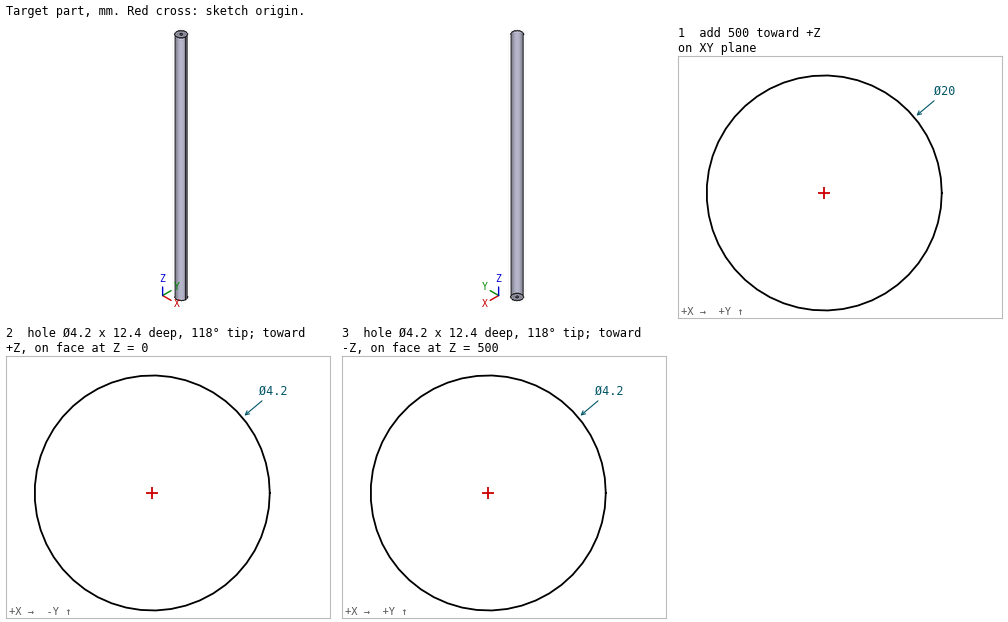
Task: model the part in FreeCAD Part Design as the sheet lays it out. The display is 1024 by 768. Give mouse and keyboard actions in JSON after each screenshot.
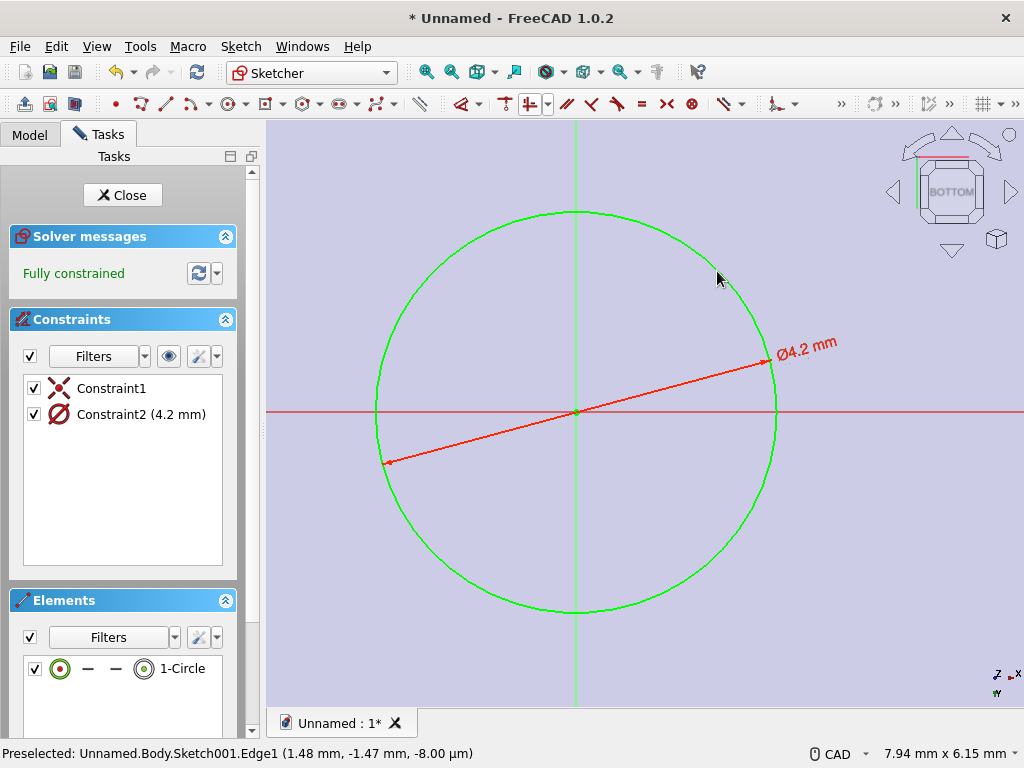
{"action": "left_click", "coordinate": [123, 195]}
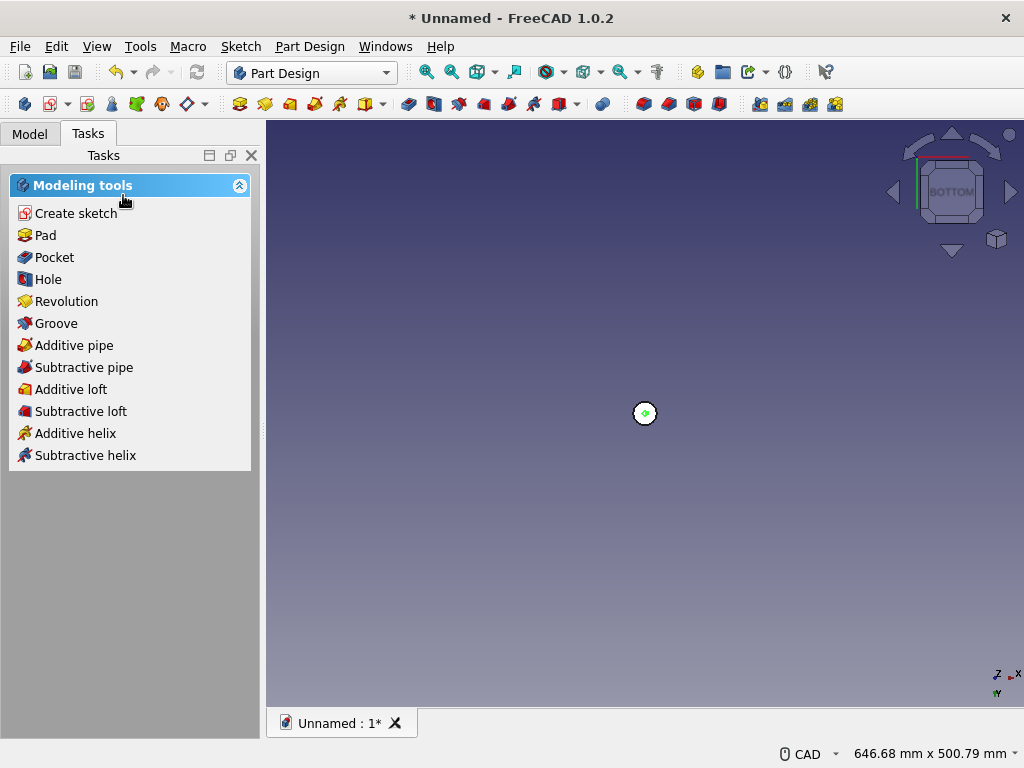
{"action": "left_click", "coordinate": [434, 104]}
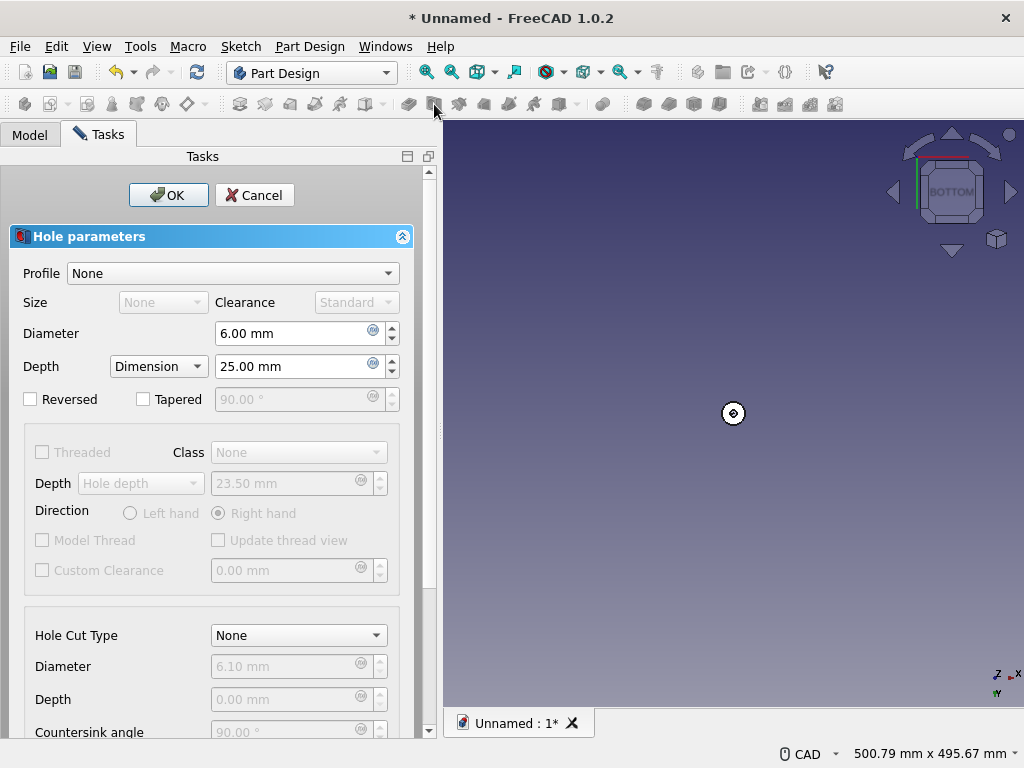
{"action": "triple_click", "coordinate": [300, 334]}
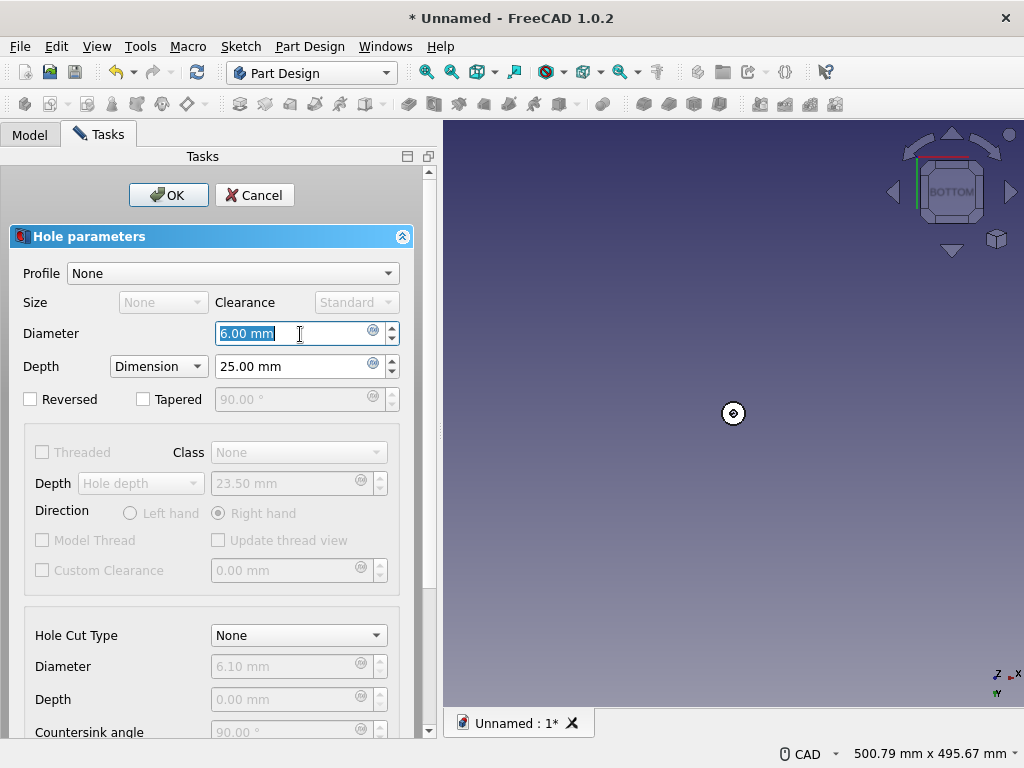
{"action": "type", "text": "4.2"}
{"action": "key", "text": "Tab"}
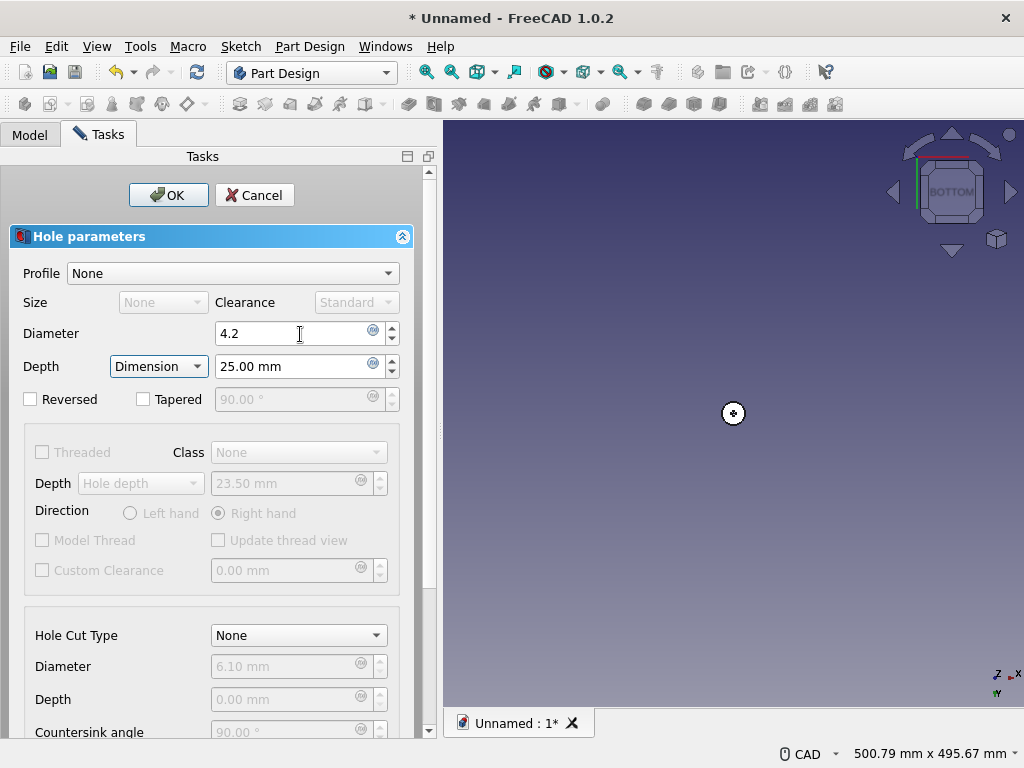
{"action": "triple_click", "coordinate": [300, 366]}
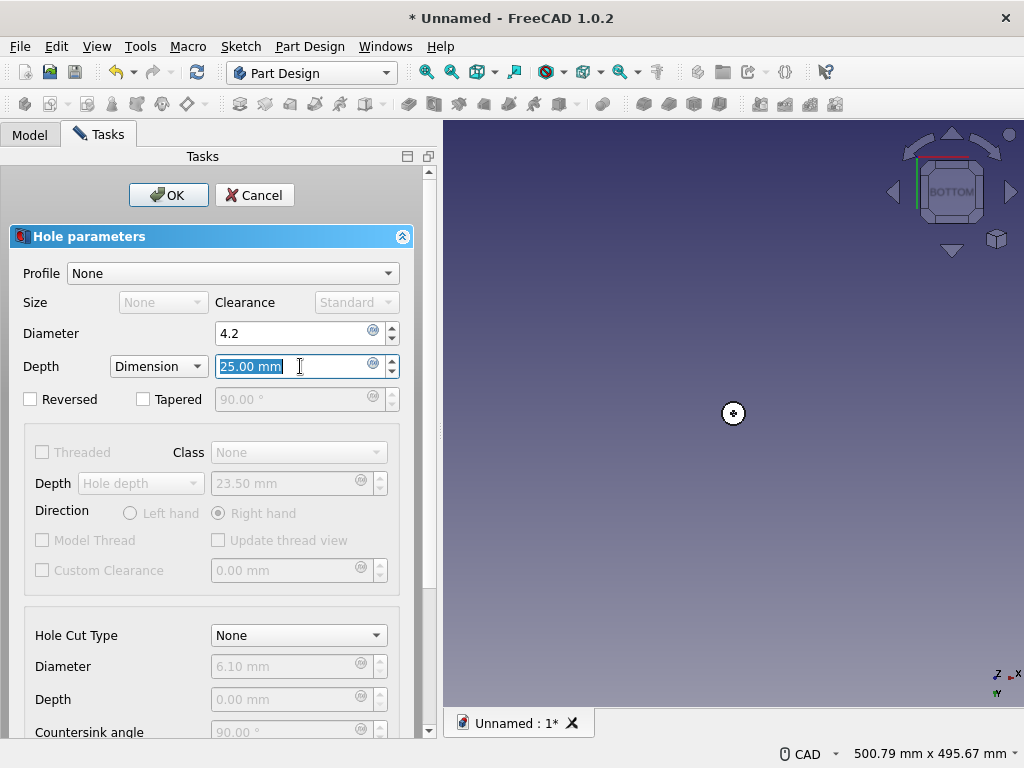
{"action": "type", "text": "12.4"}
{"action": "key", "text": "Tab"}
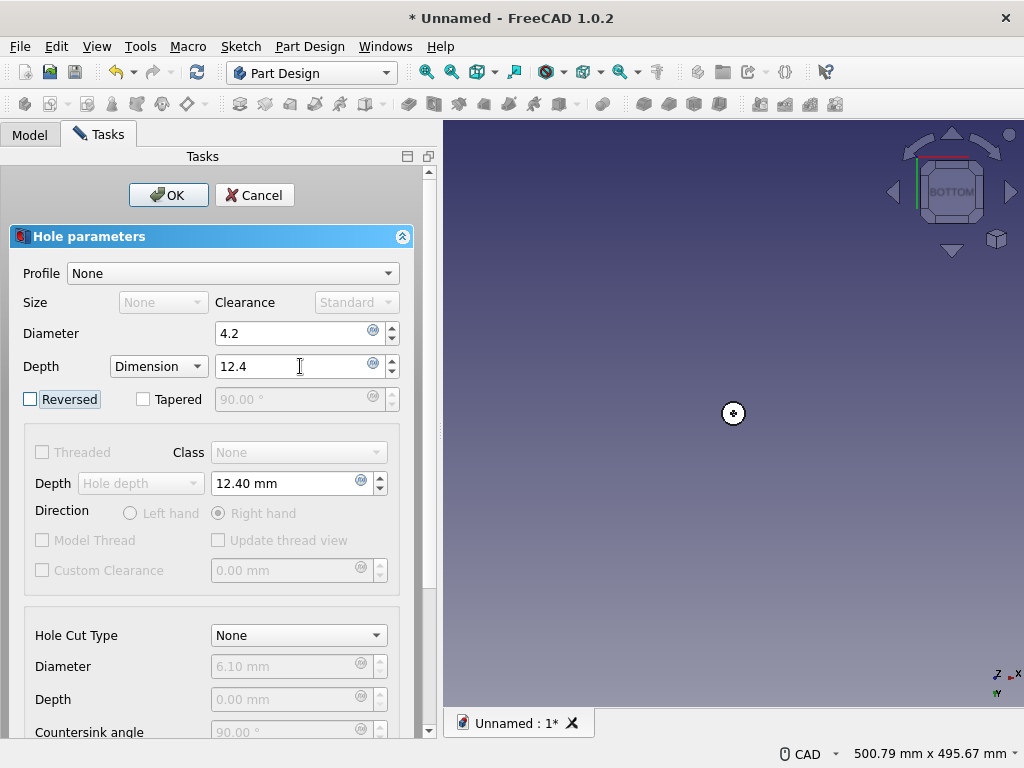
{"action": "left_click", "coordinate": [169, 195]}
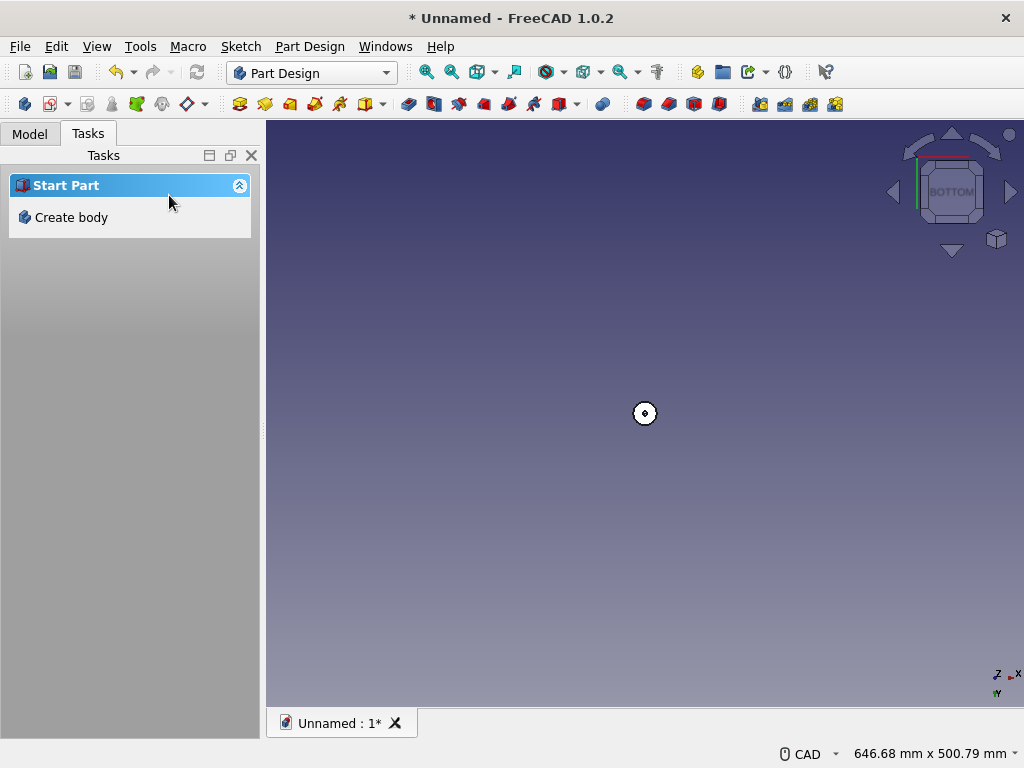
{"action": "left_click", "coordinate": [427, 72]}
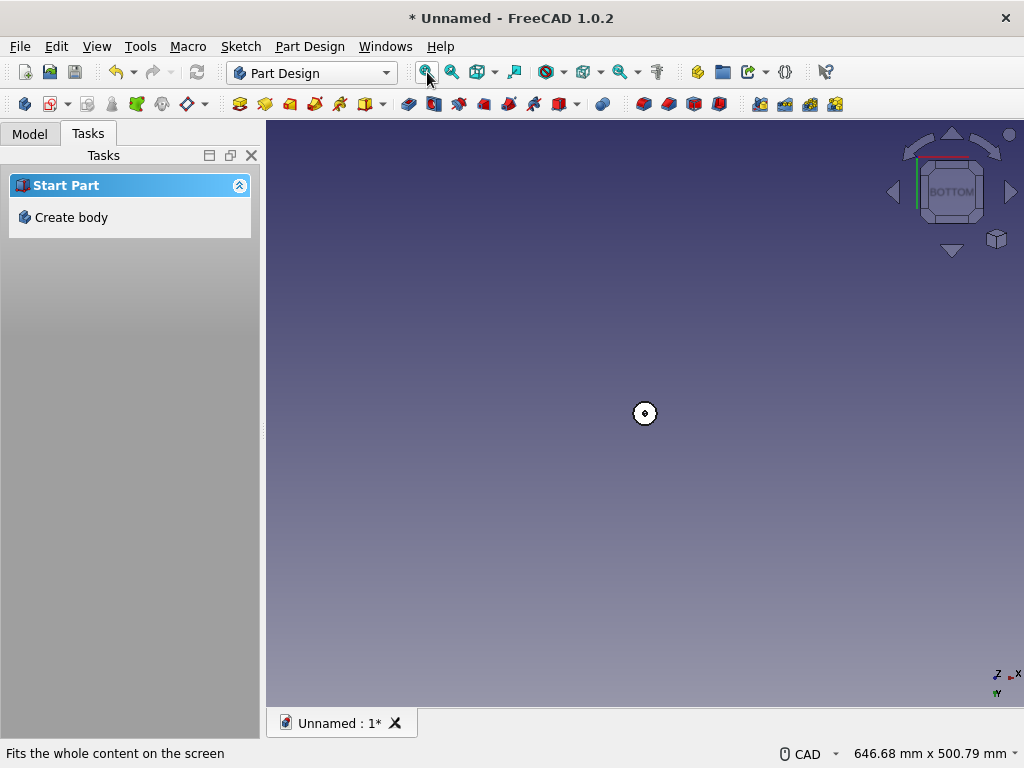
{"action": "key", "text": "0"}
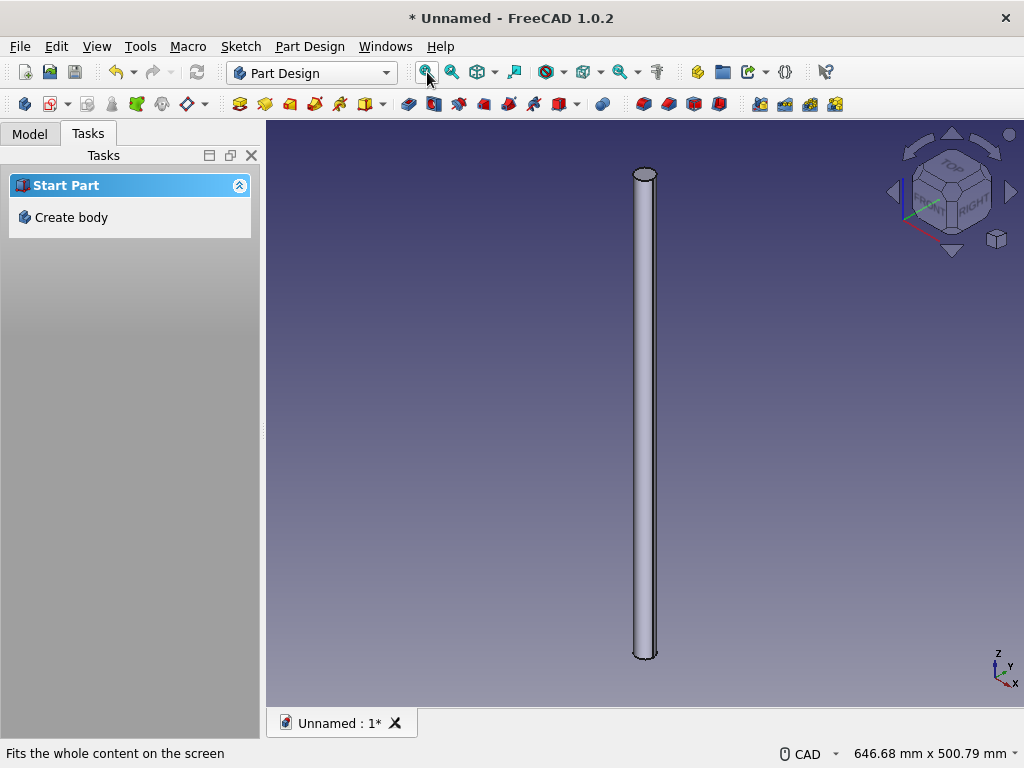
{"action": "key", "text": "2"}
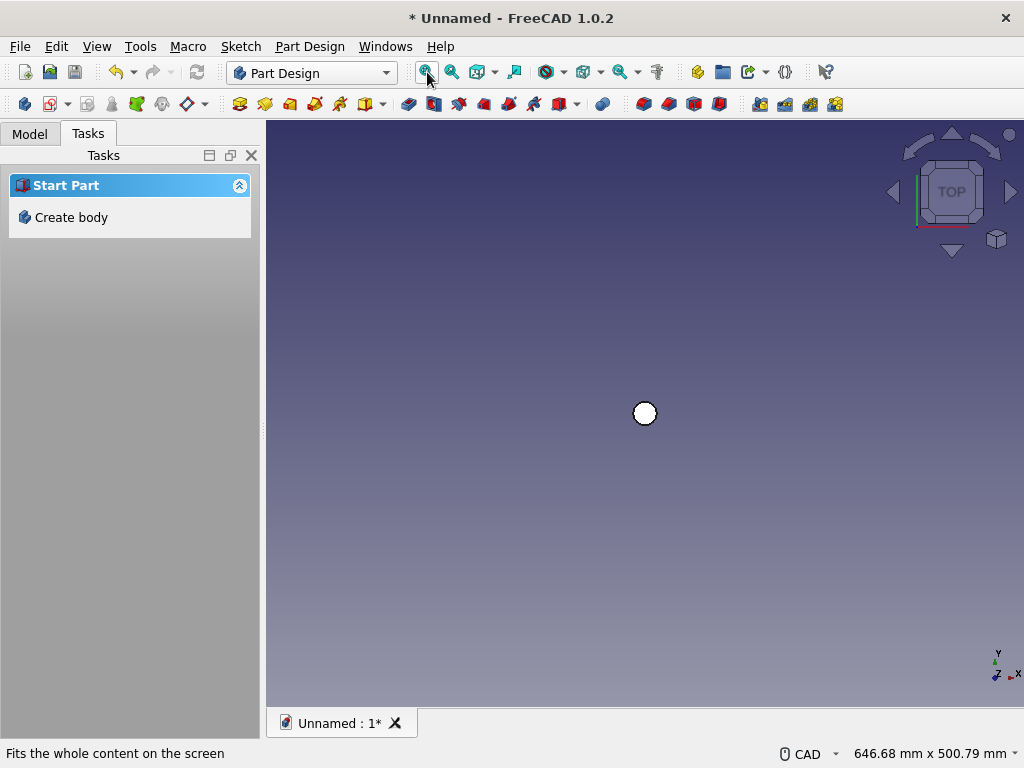
{"action": "left_click", "coordinate": [427, 72]}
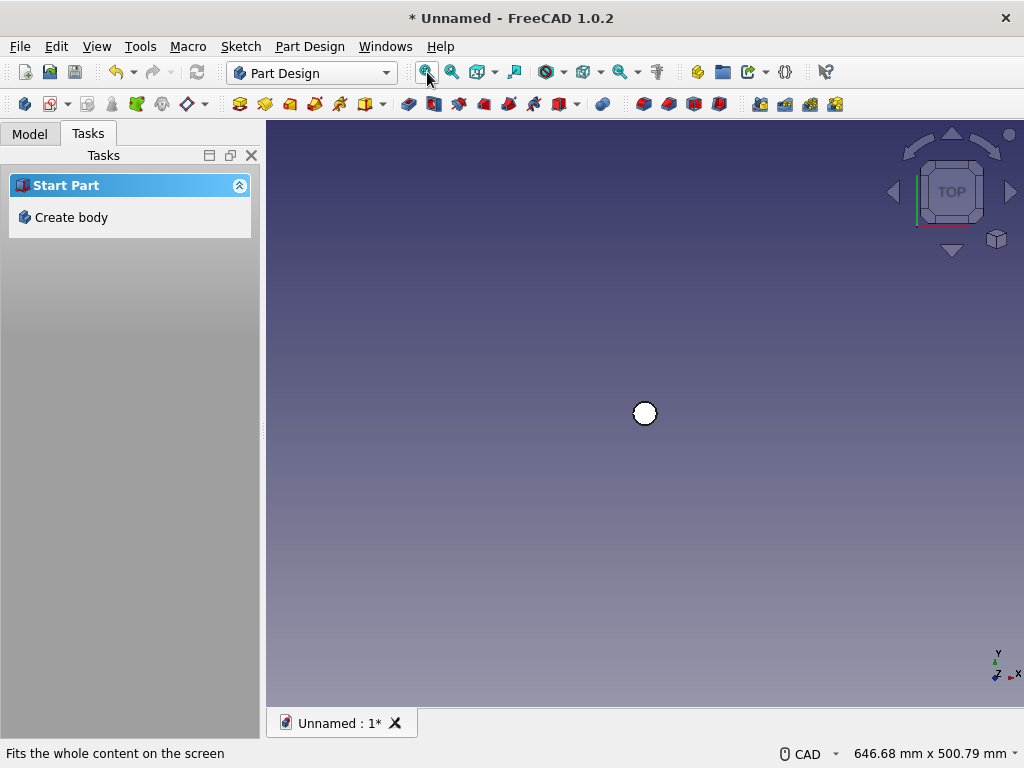
{"action": "left_click", "coordinate": [645, 412]}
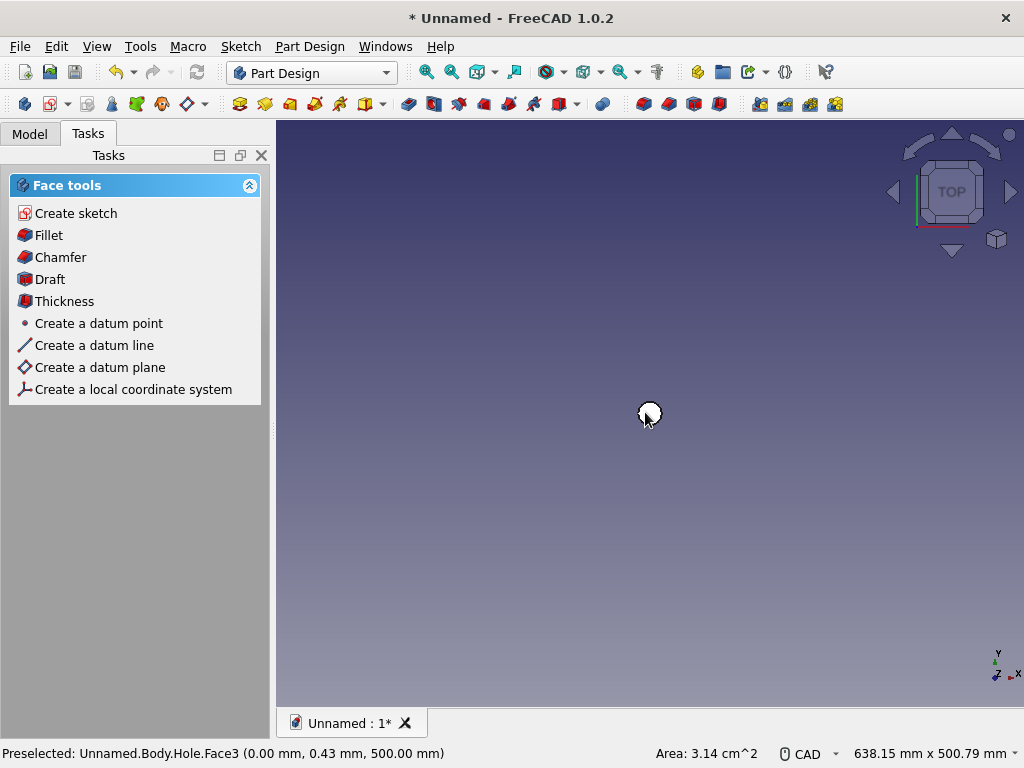
{"action": "left_click", "coordinate": [50, 104]}